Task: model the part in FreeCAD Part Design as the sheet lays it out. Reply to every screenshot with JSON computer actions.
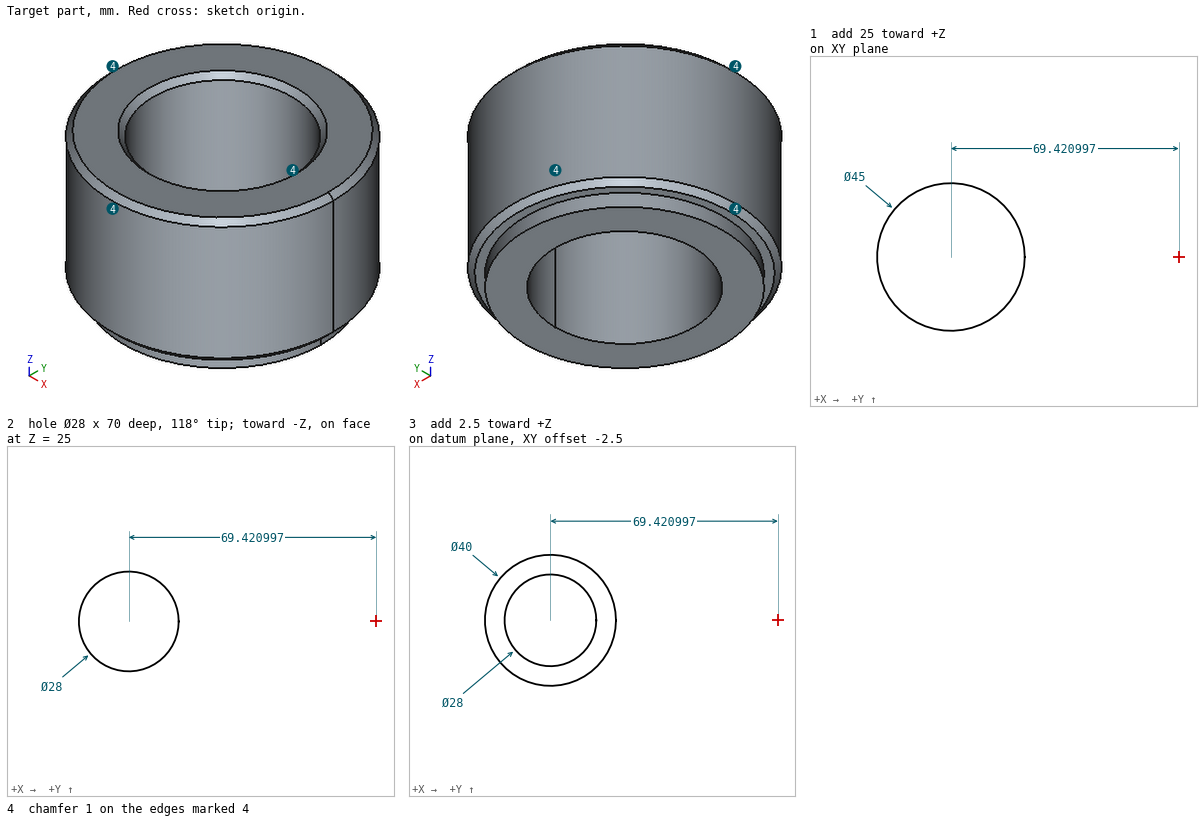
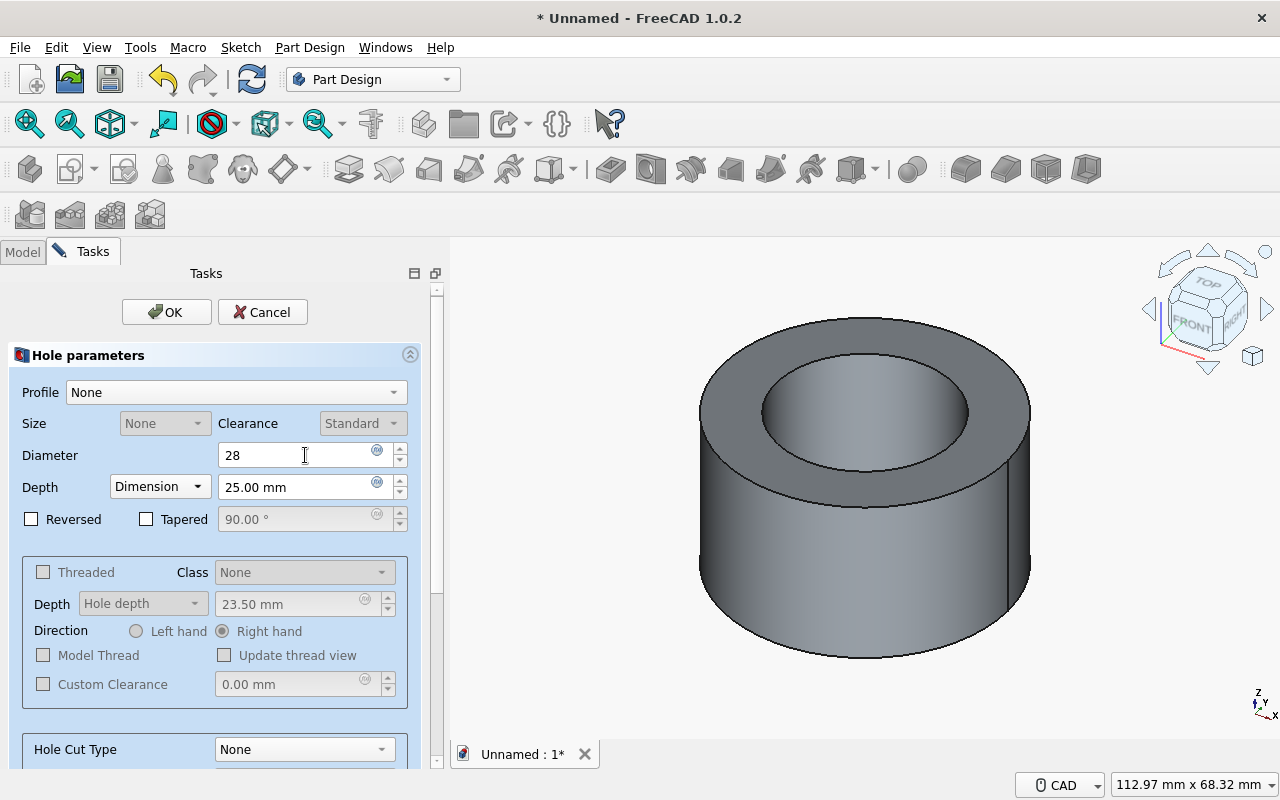
{"action": "triple_click", "coordinate": [305, 487]}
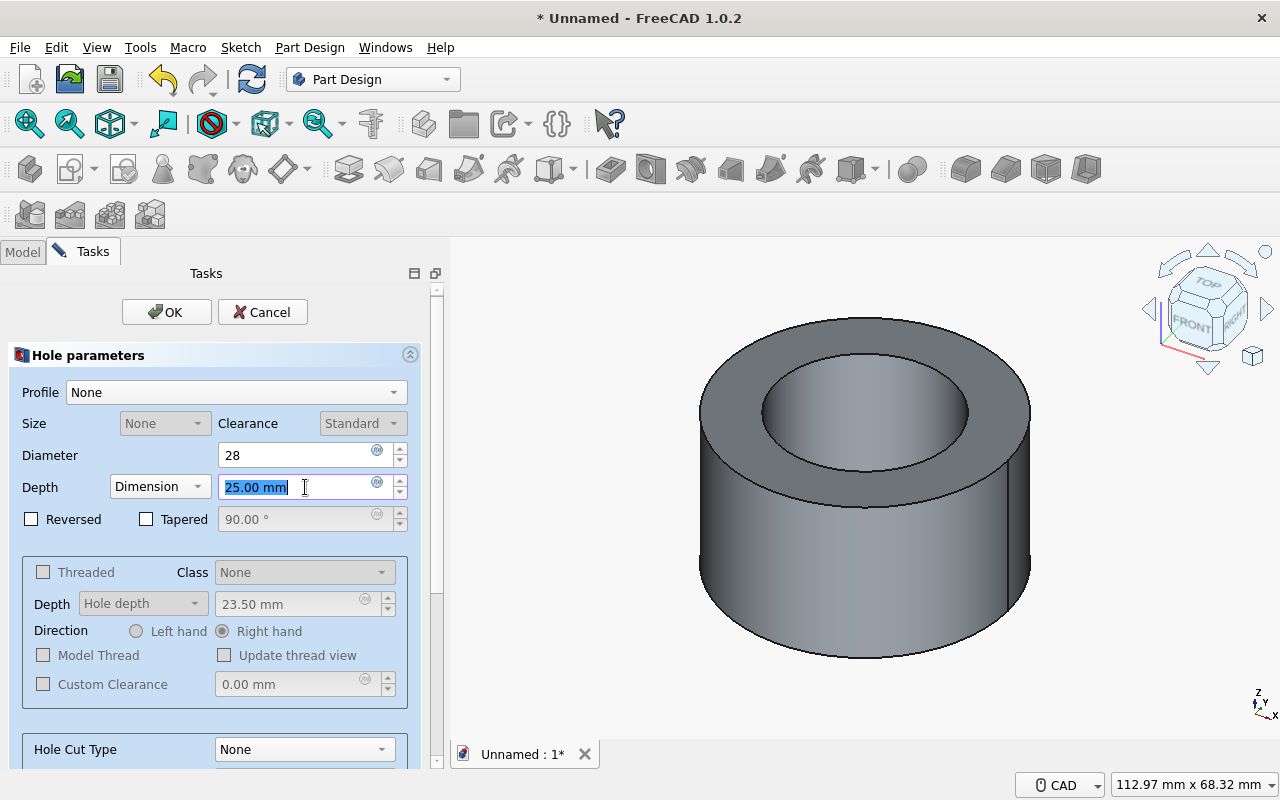
{"action": "type", "text": "70"}
{"action": "key", "text": "Tab"}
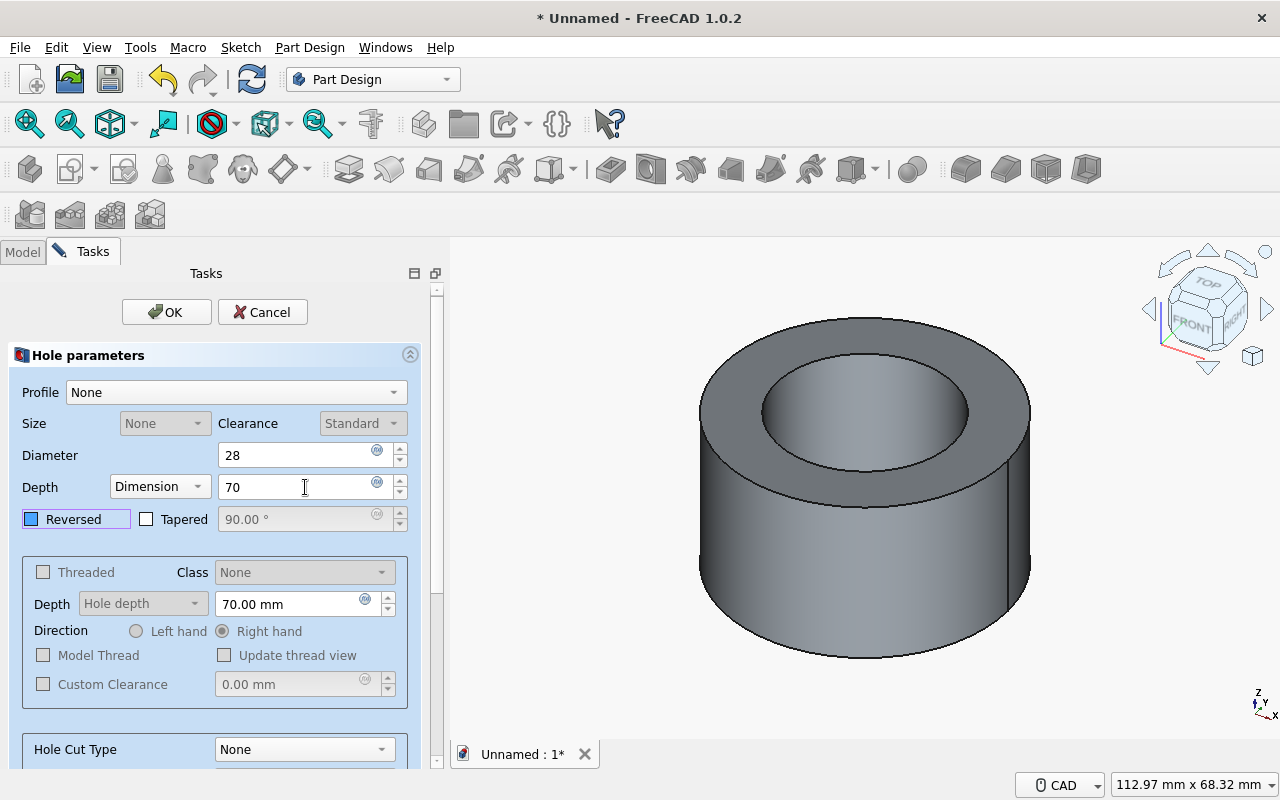
{"action": "left_click", "coordinate": [167, 312]}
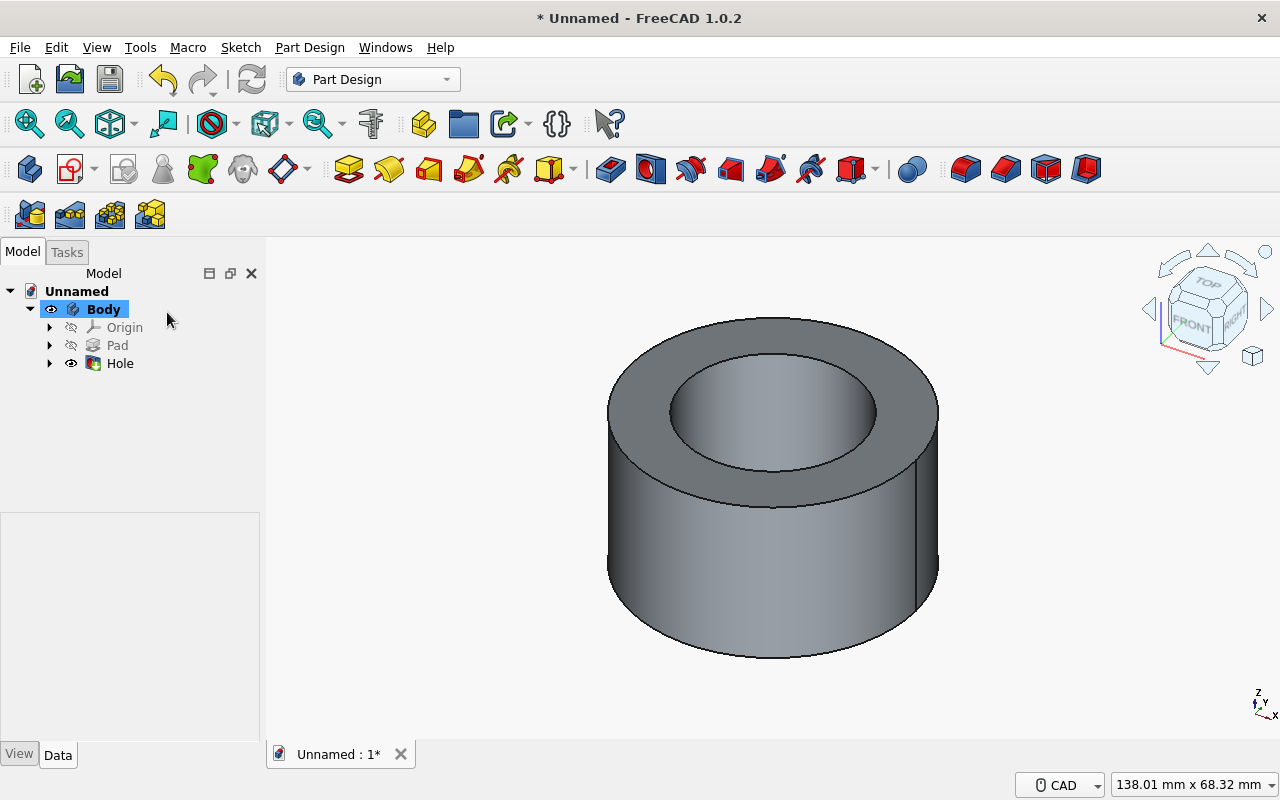
{"action": "left_click", "coordinate": [50, 327]}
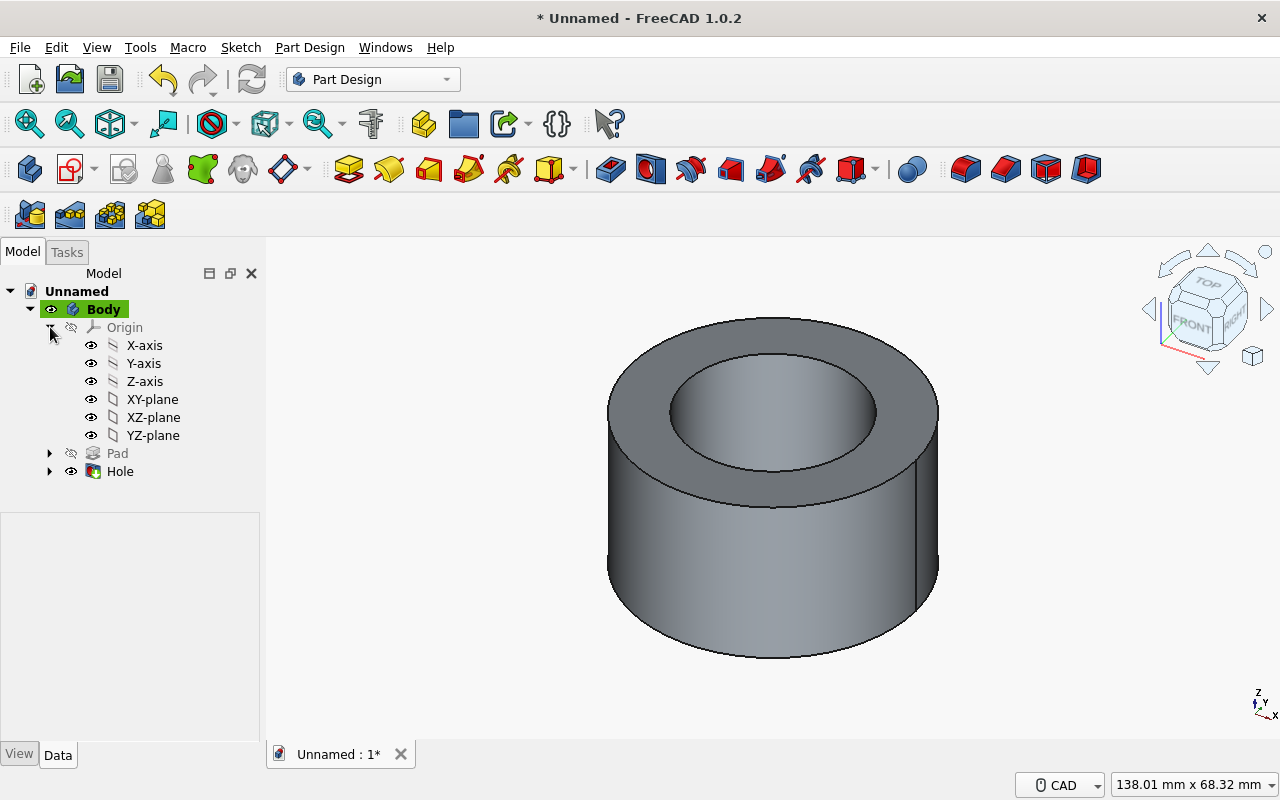
{"action": "left_click", "coordinate": [136, 399]}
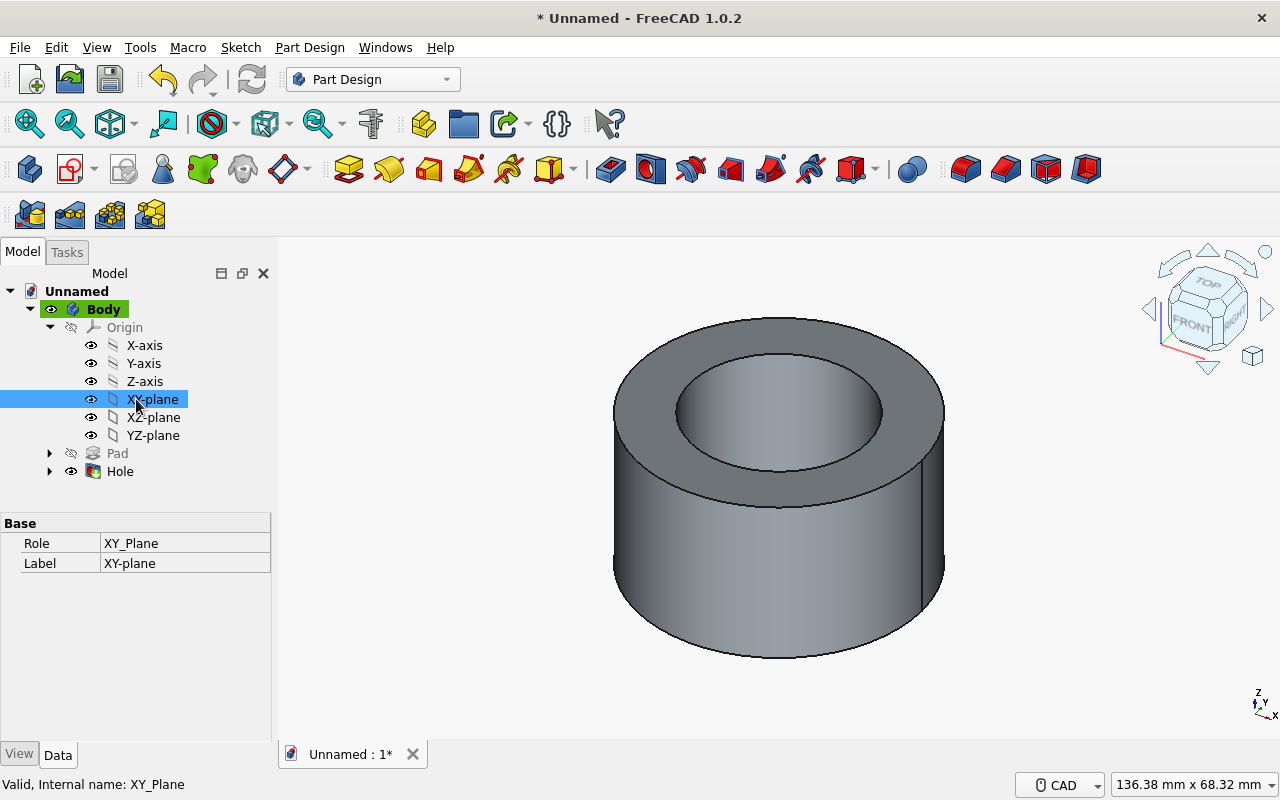
{"action": "left_click", "coordinate": [284, 170]}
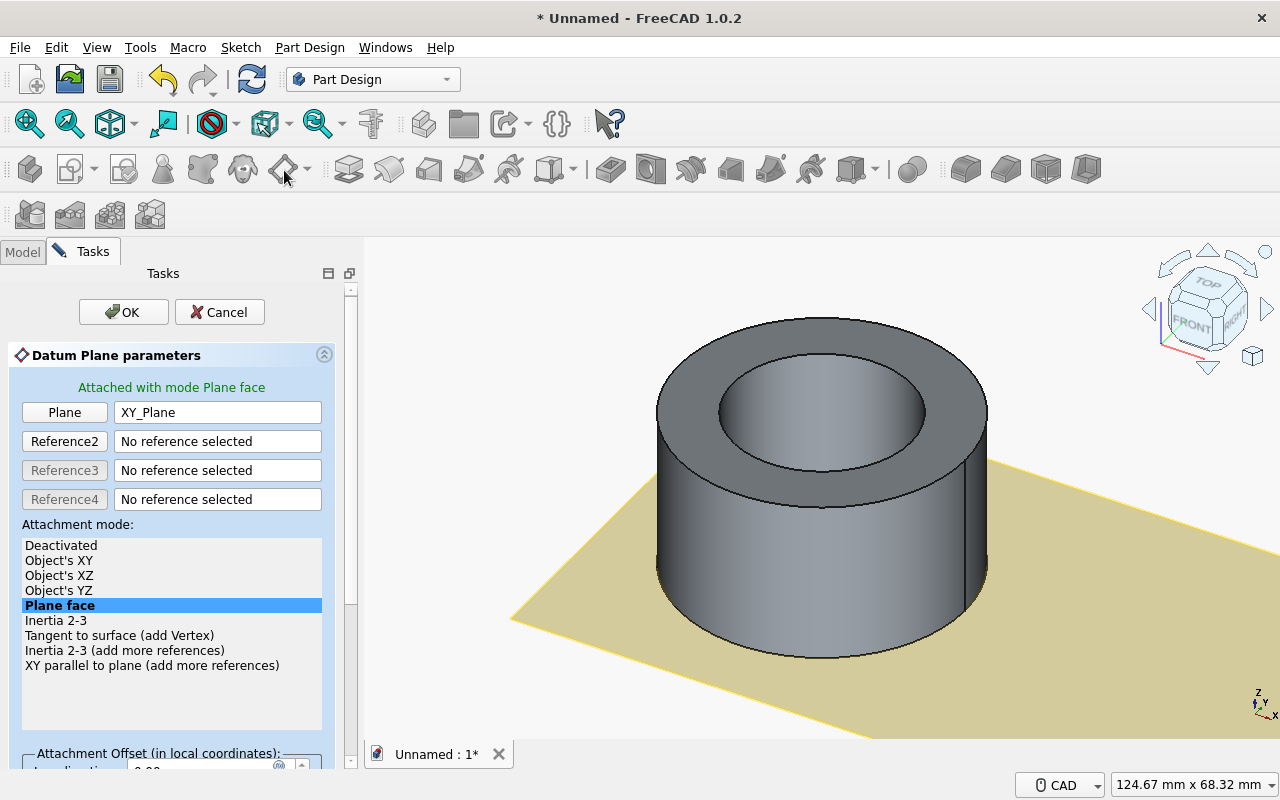
{"action": "scroll", "coordinate": [351, 526], "scroll_direction": "down", "scroll_amount": 3}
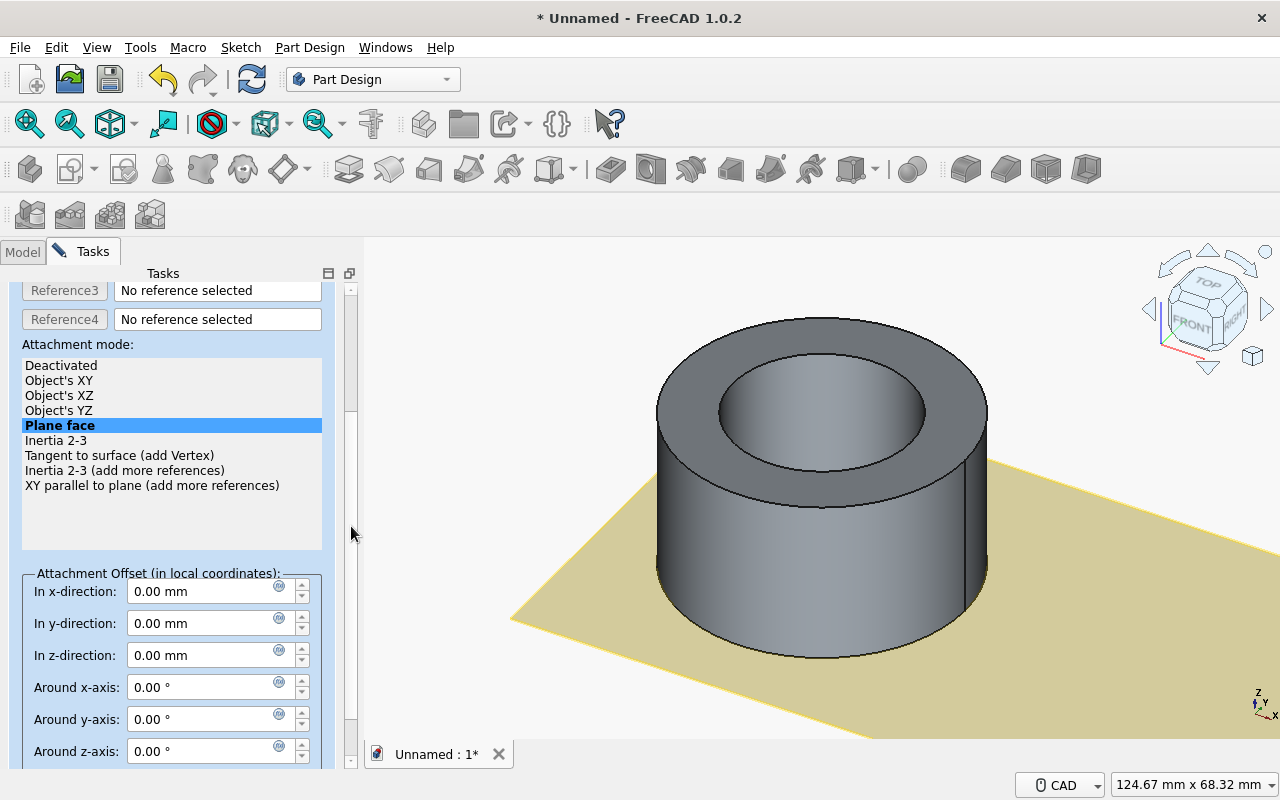
{"action": "triple_click", "coordinate": [210, 655]}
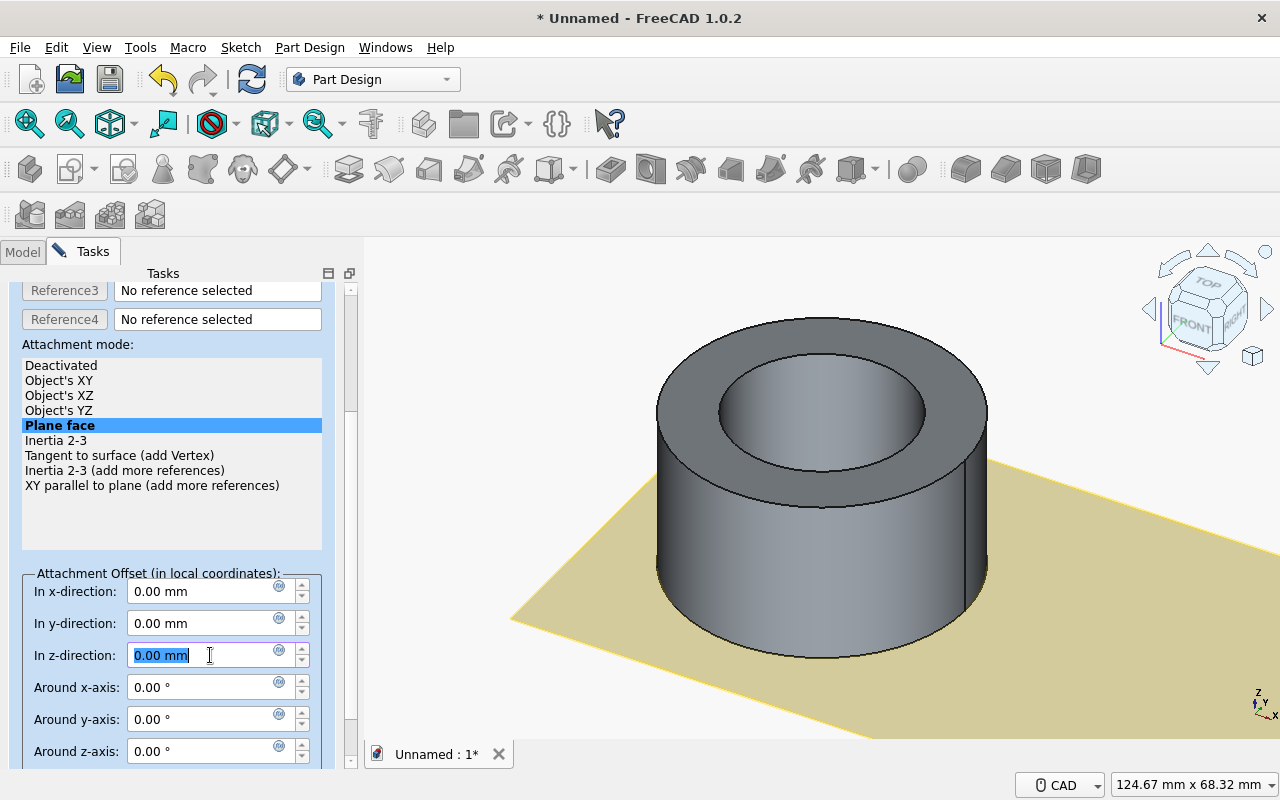
{"action": "type", "text": "-2.5"}
{"action": "key", "text": "Tab"}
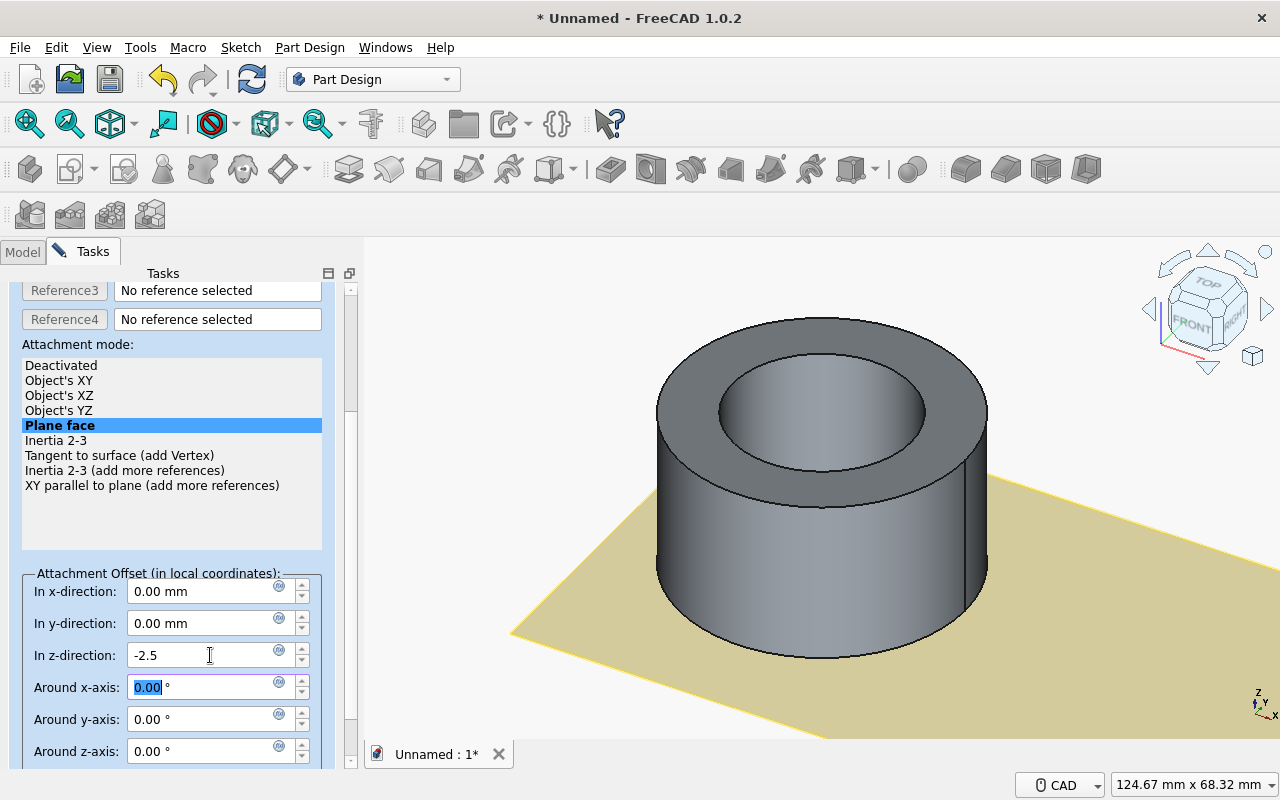
{"action": "scroll", "coordinate": [351, 526], "scroll_direction": "up", "scroll_amount": 4}